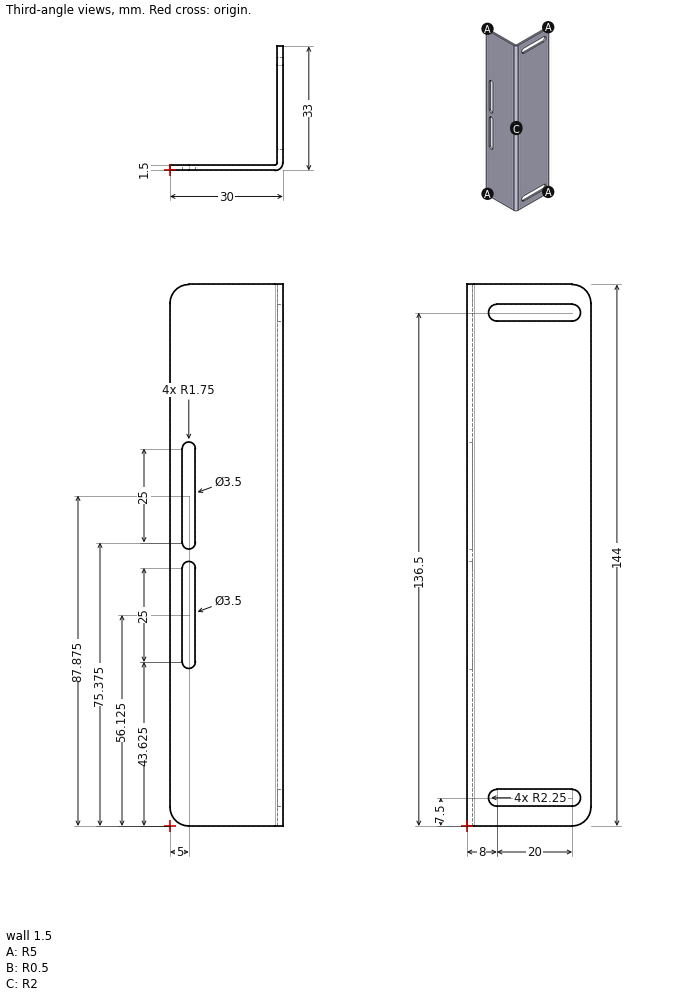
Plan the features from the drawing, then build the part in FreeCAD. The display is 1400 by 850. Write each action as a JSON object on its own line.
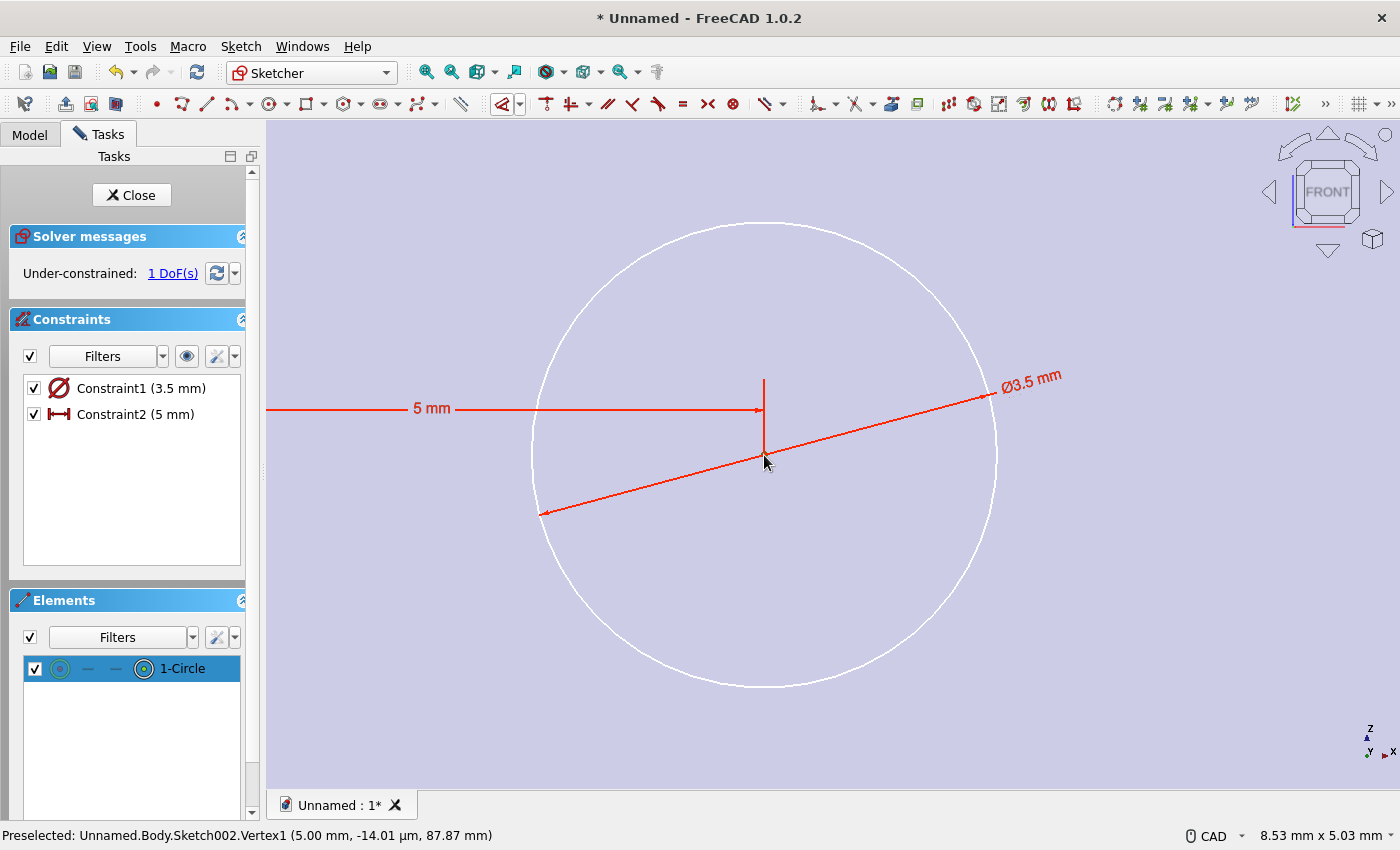
{"action": "key", "text": "i"}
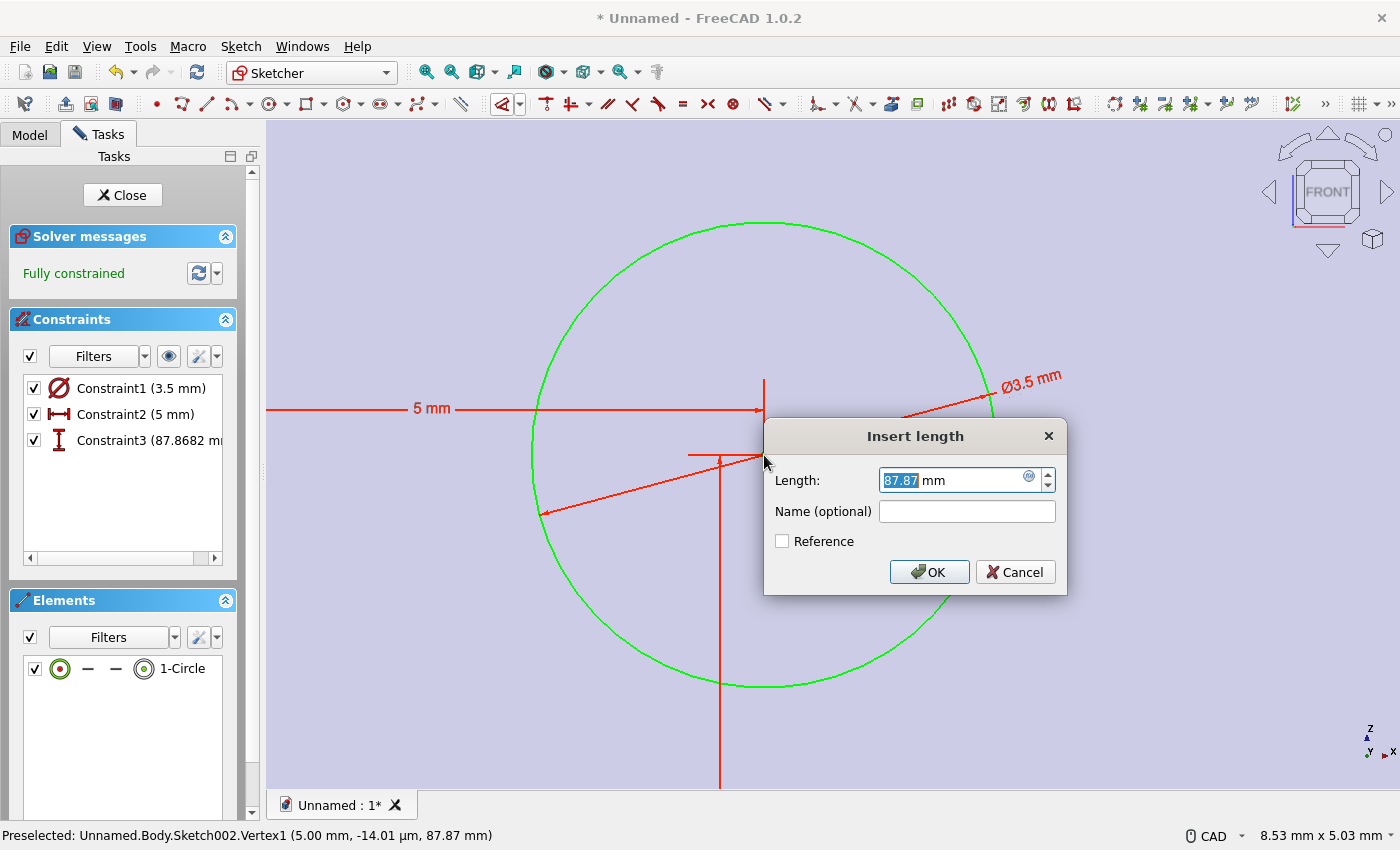
{"action": "type", "text": "87.875"}
{"action": "key", "text": "Return"}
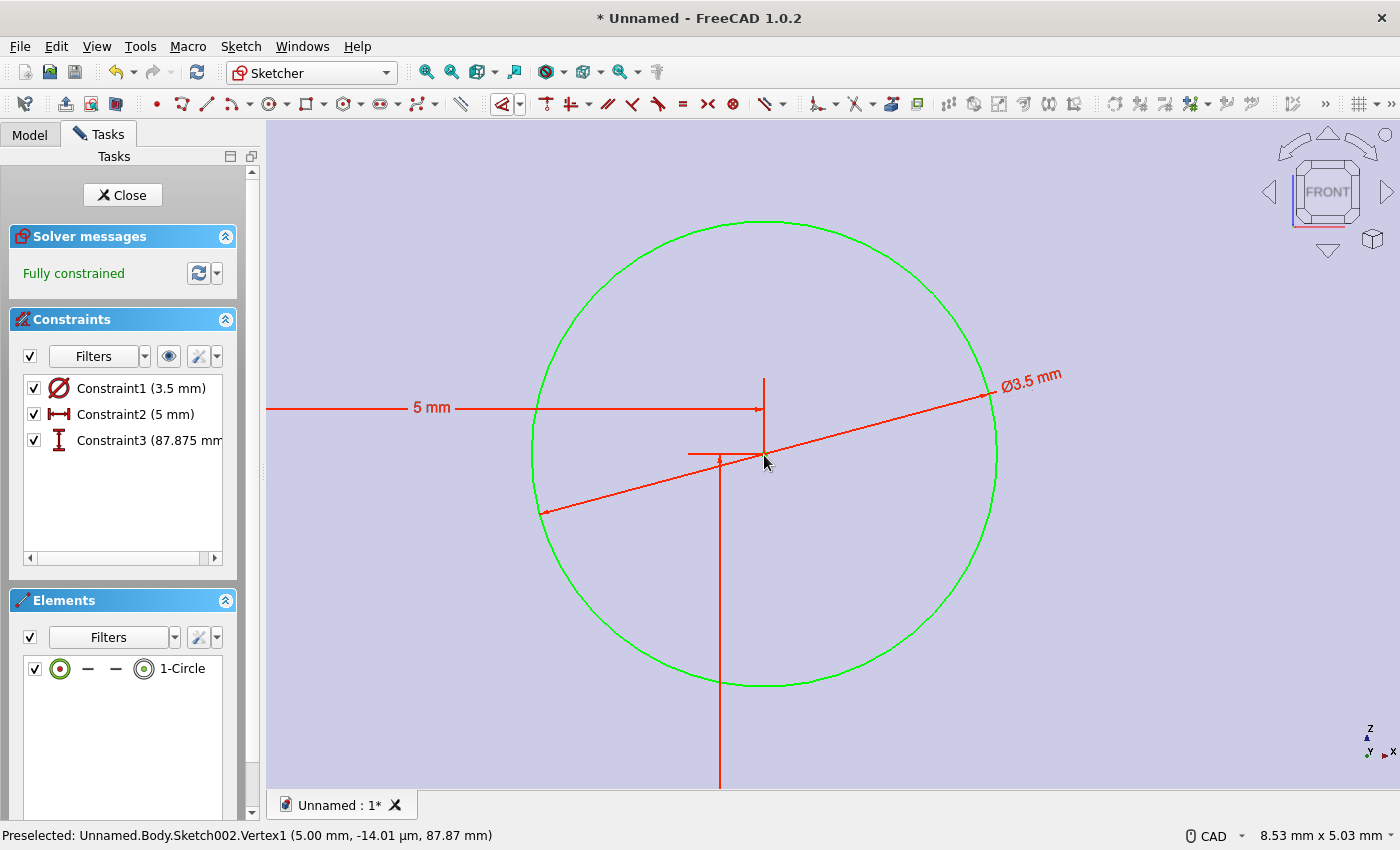
{"action": "left_click", "coordinate": [123, 195]}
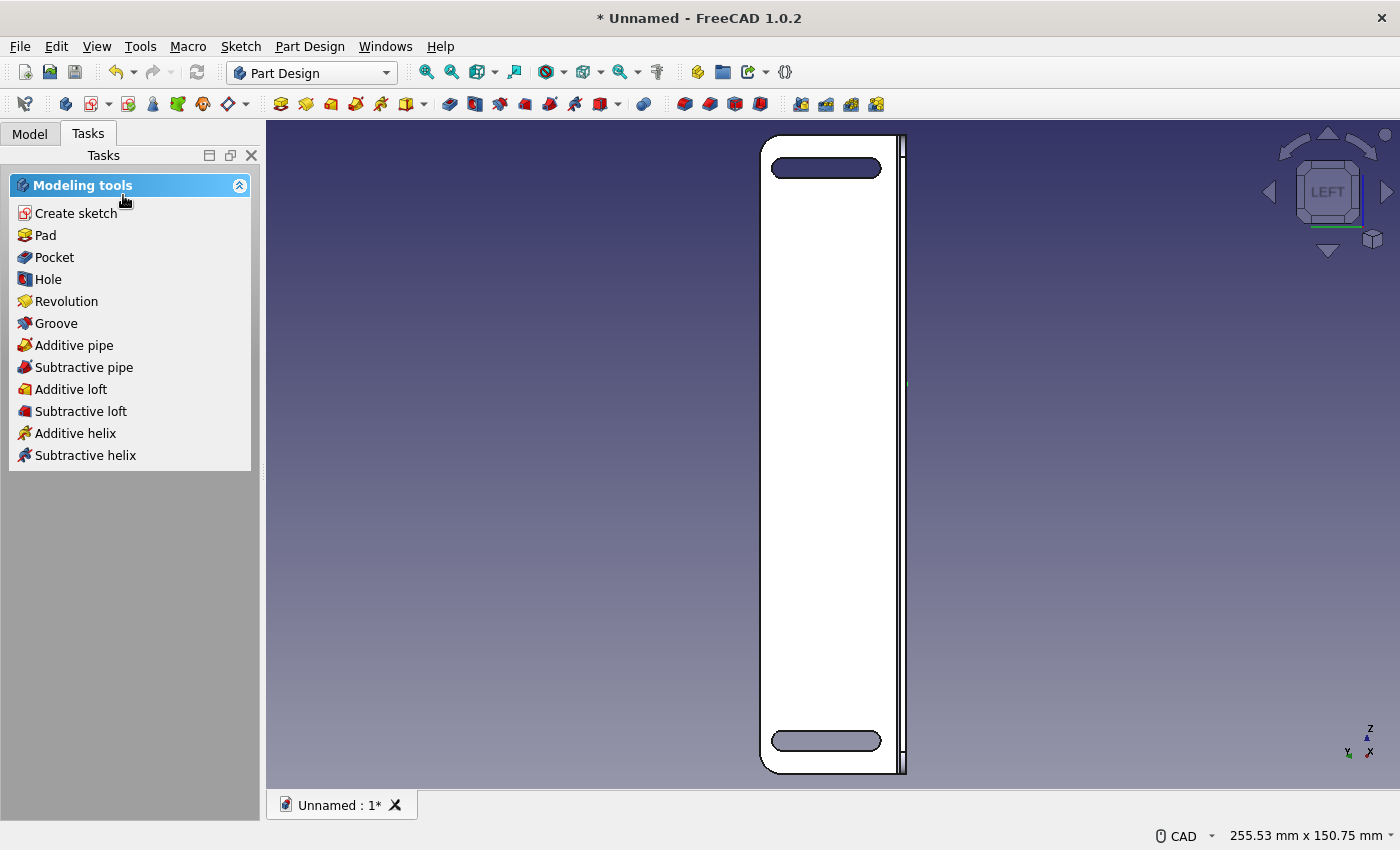
{"action": "left_click", "coordinate": [450, 104]}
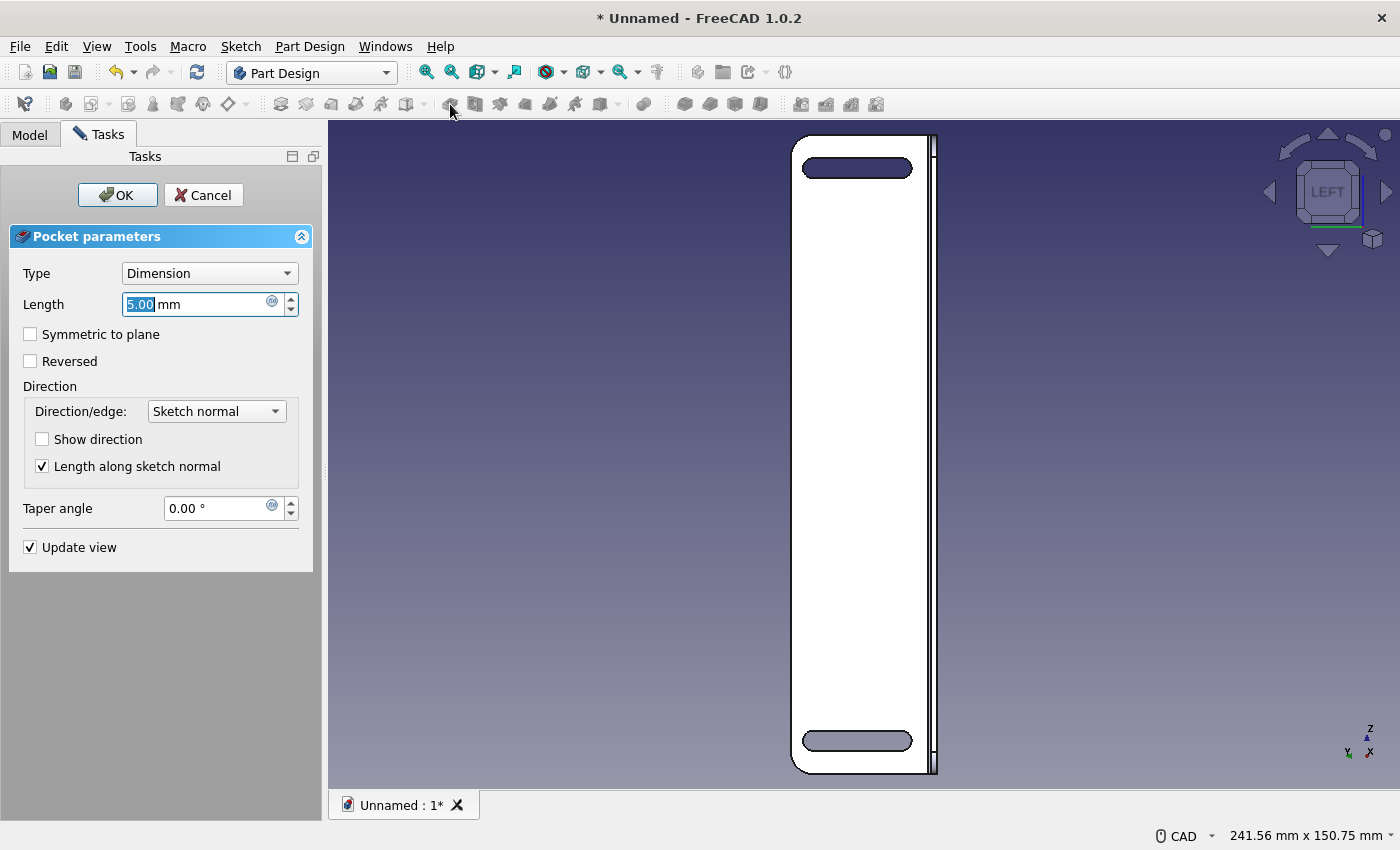
{"action": "left_click", "coordinate": [210, 274]}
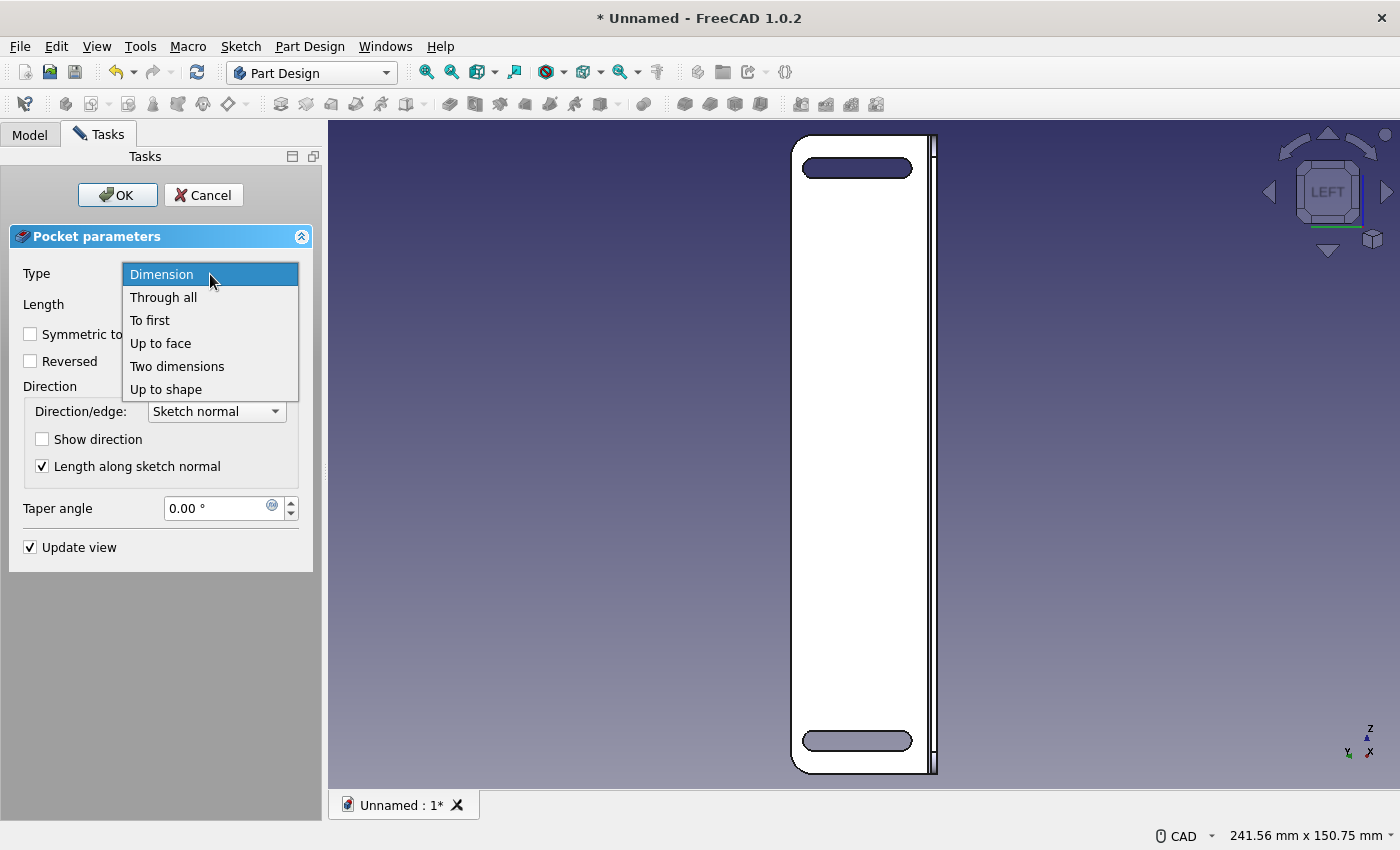
{"action": "left_click", "coordinate": [208, 320]}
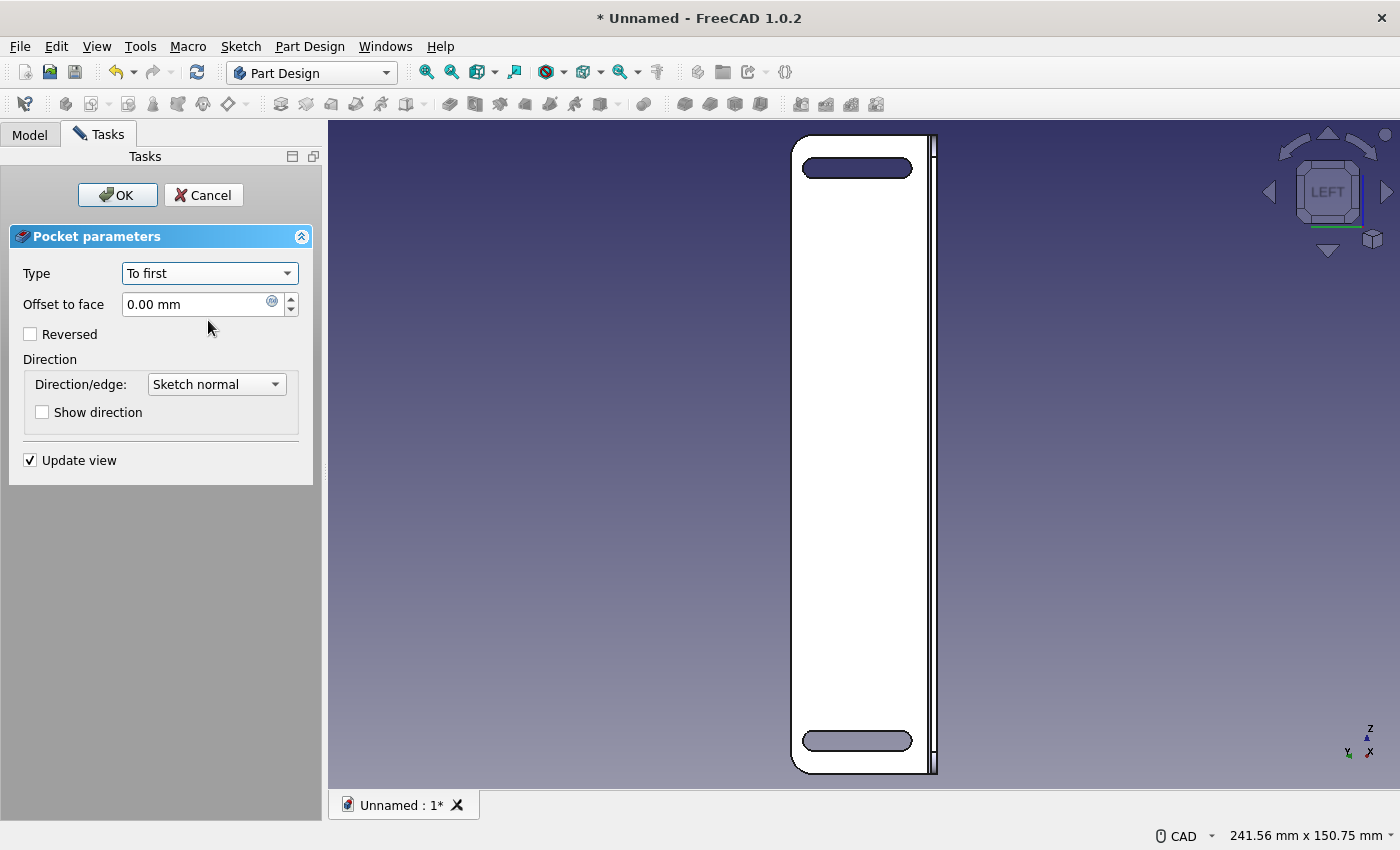
{"action": "left_click", "coordinate": [118, 195]}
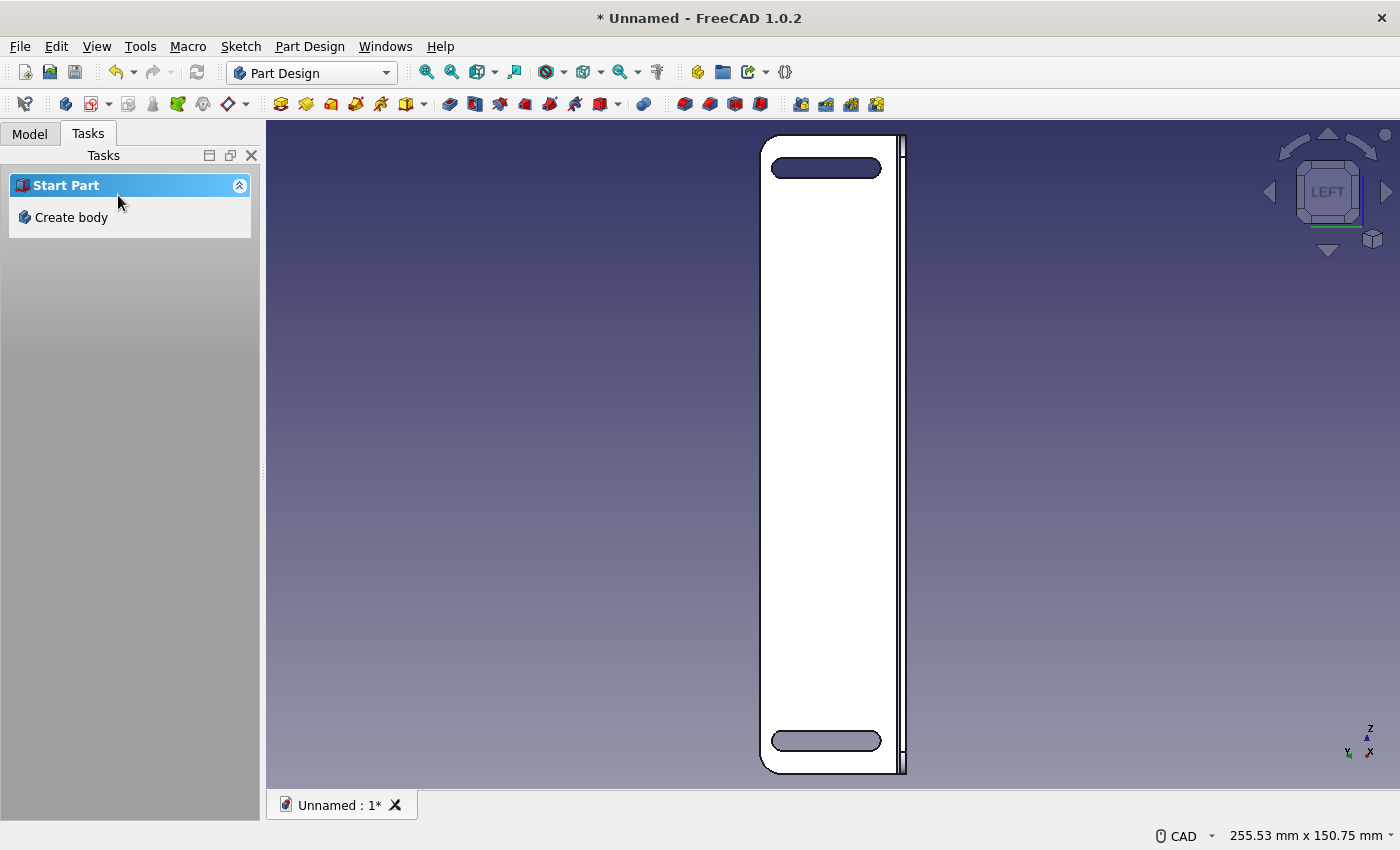
{"action": "key", "text": "0"}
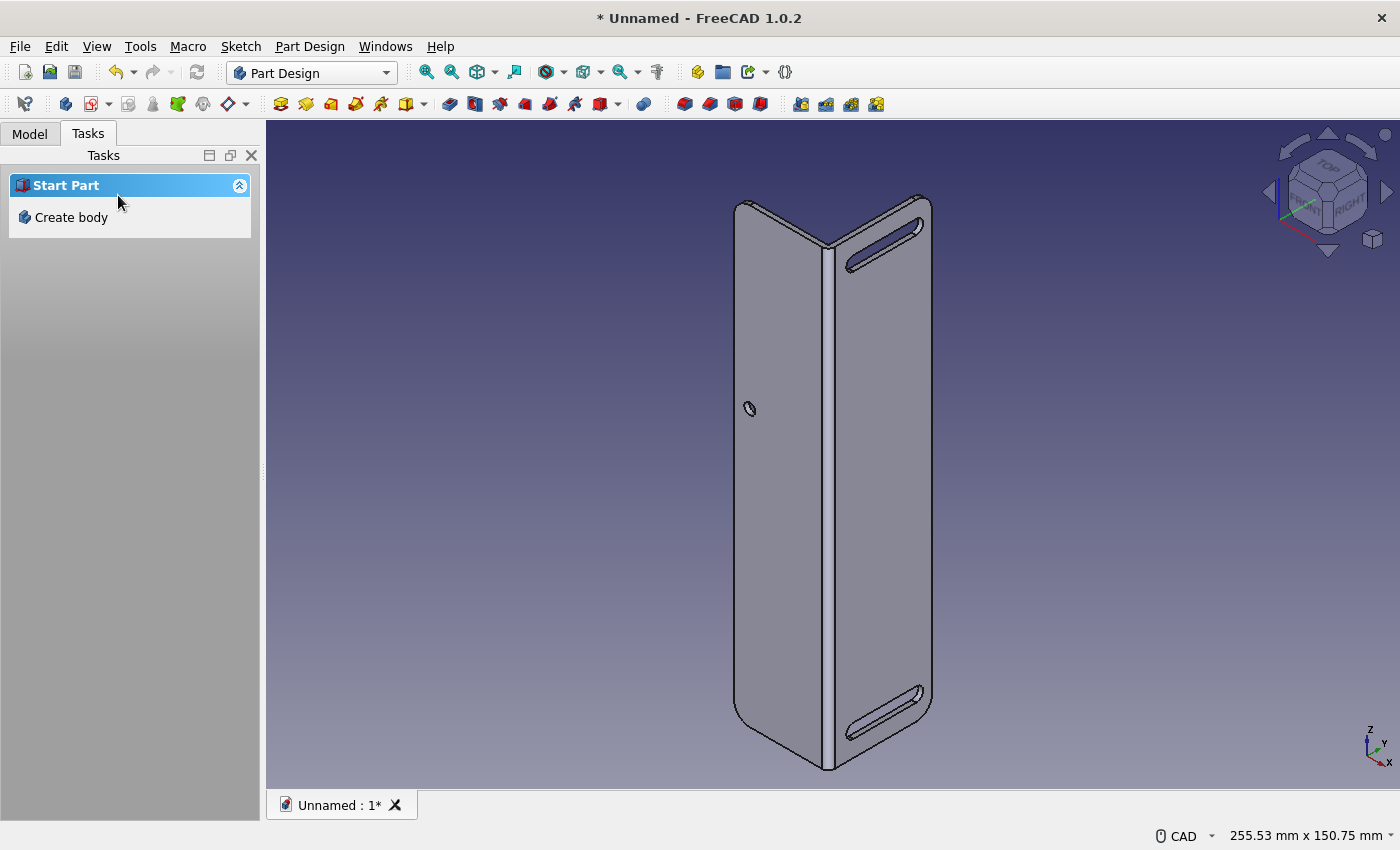
{"action": "left_click", "coordinate": [778, 333]}